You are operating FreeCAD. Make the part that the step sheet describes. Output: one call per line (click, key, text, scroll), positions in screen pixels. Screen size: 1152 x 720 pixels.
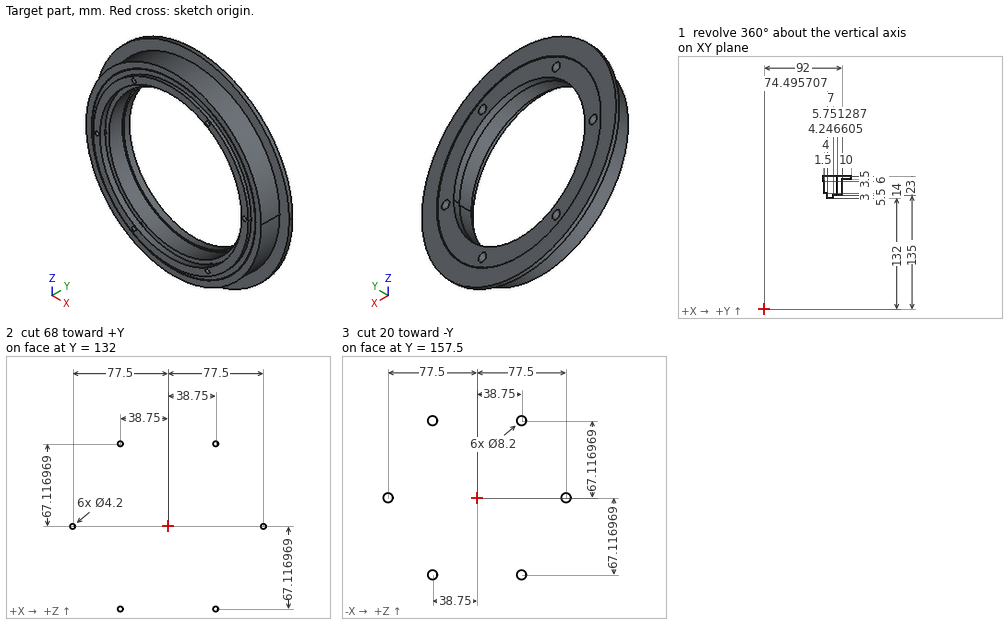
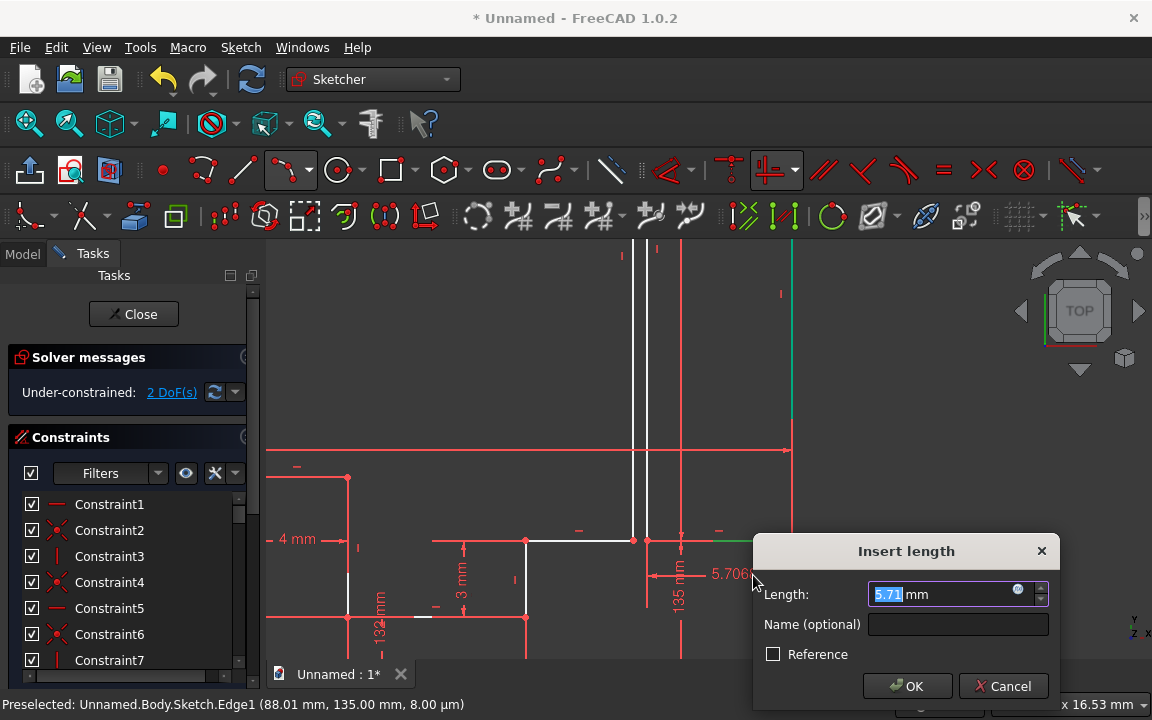
text(5.751287)
key(Return)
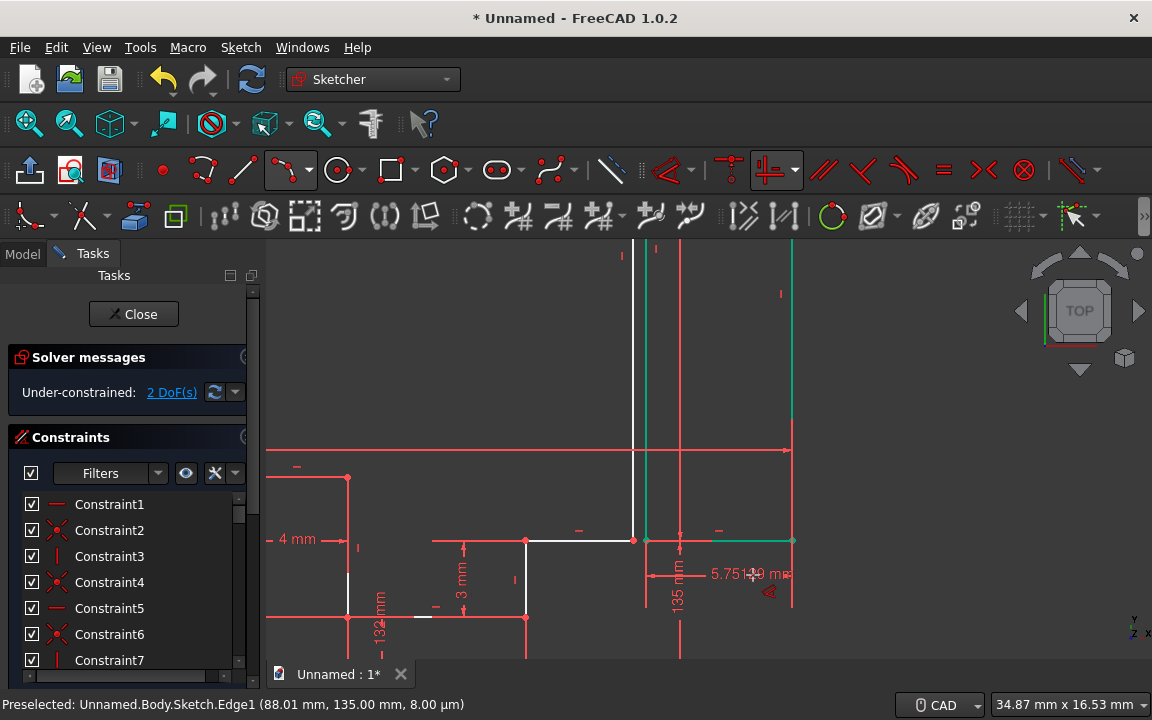
click(558, 541)
click(579, 575)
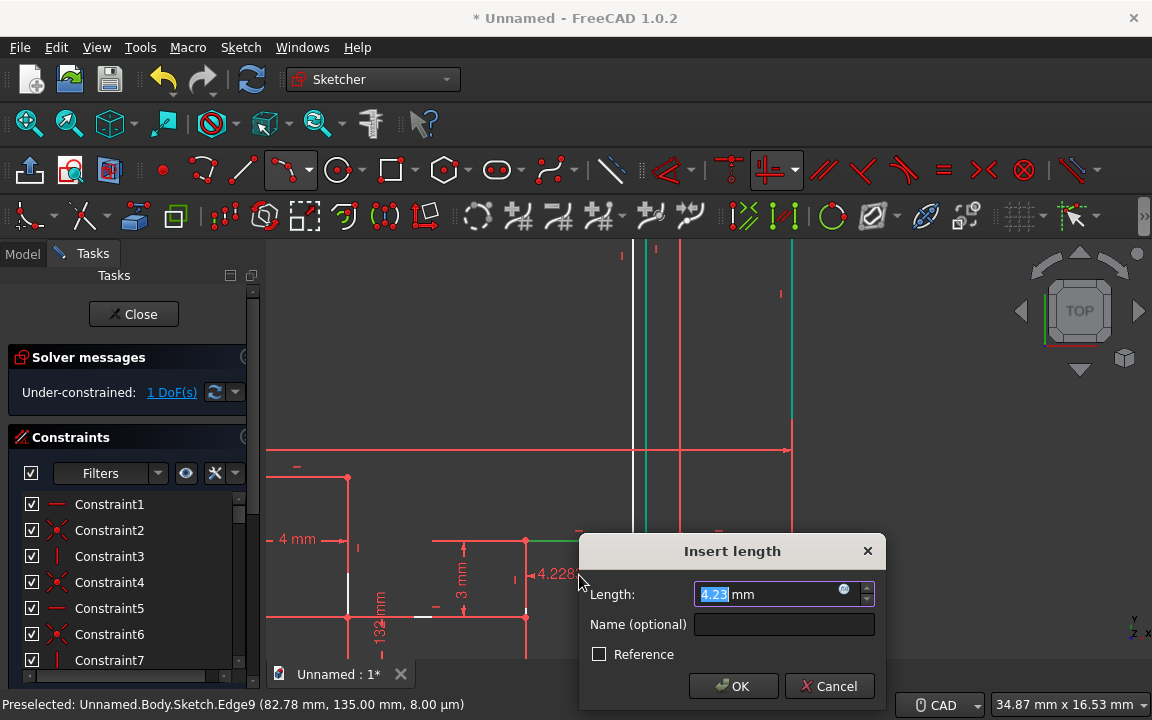
text(4.246605)
key(Return)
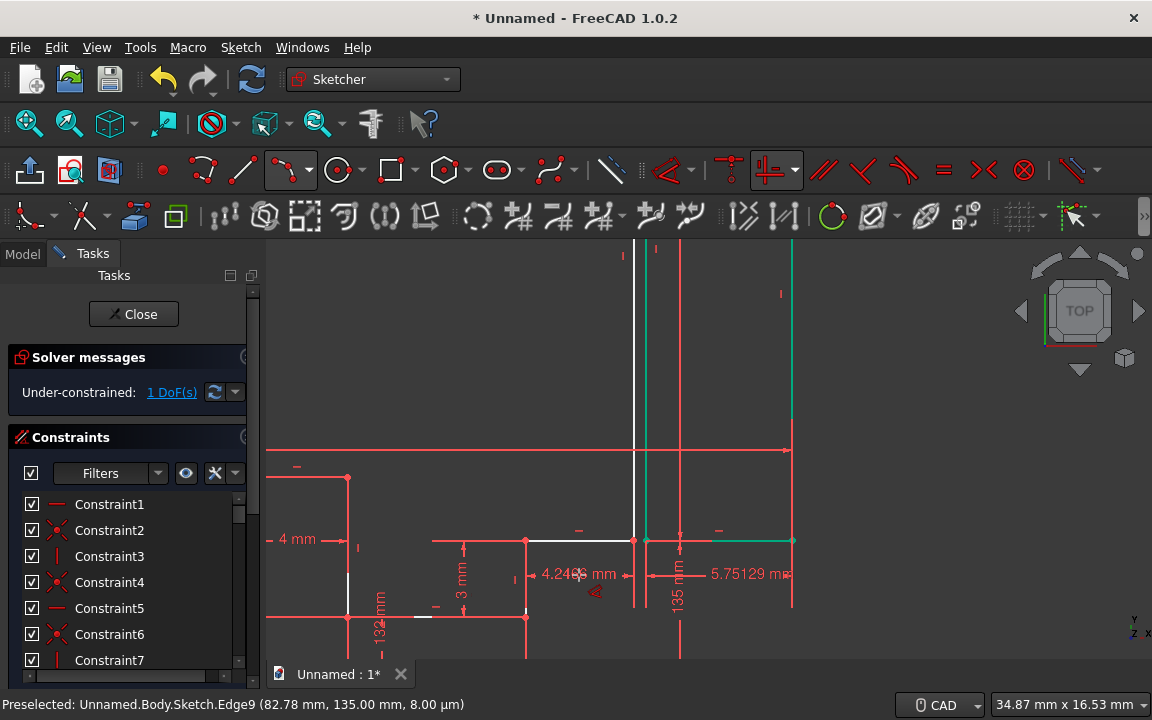
click(348, 617)
click(333, 583)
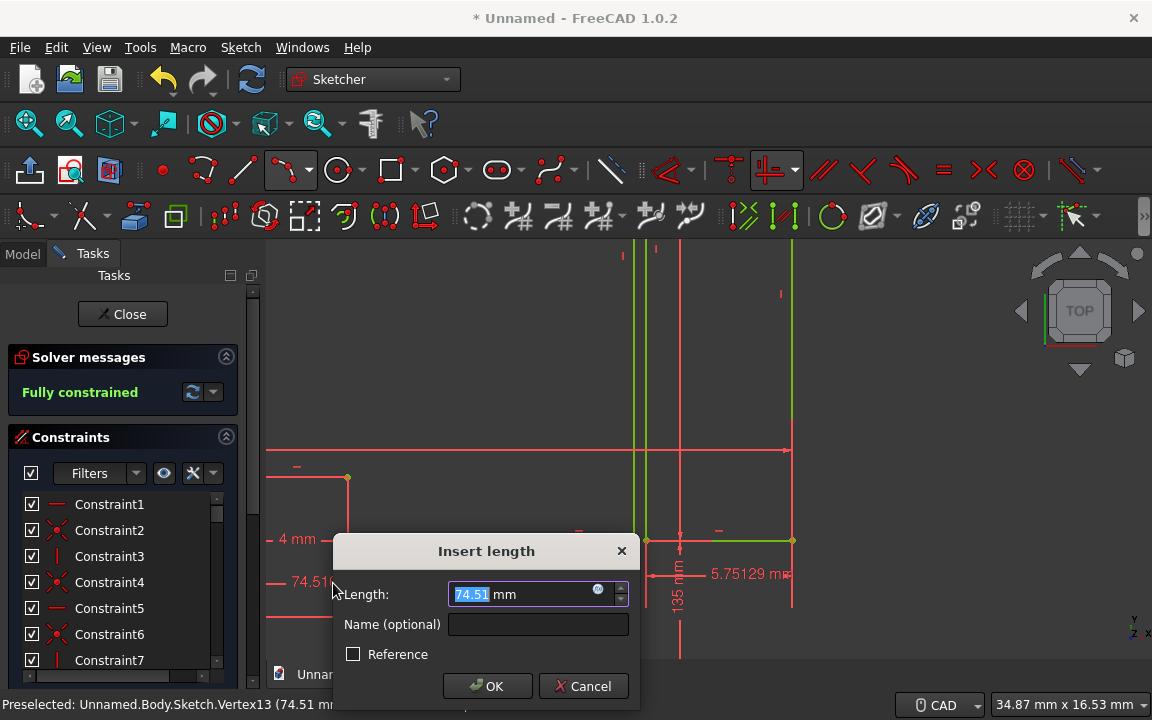
text(74.495707)
key(Return)
key(Escape)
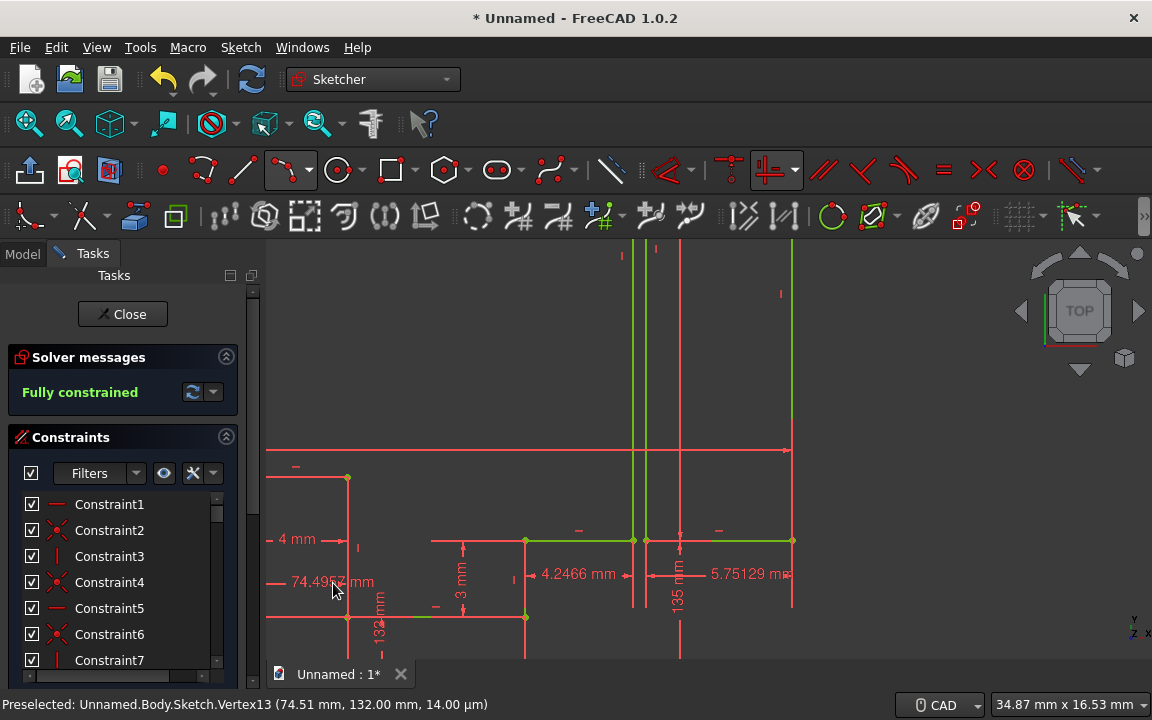
click(123, 314)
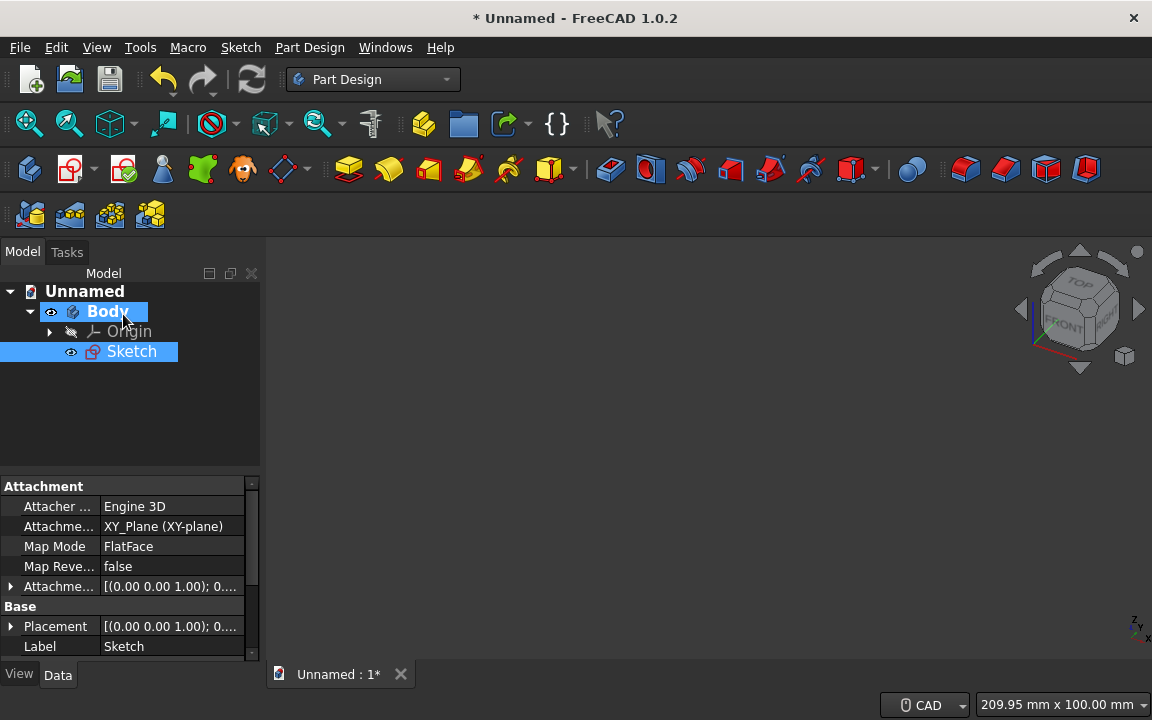
click(390, 170)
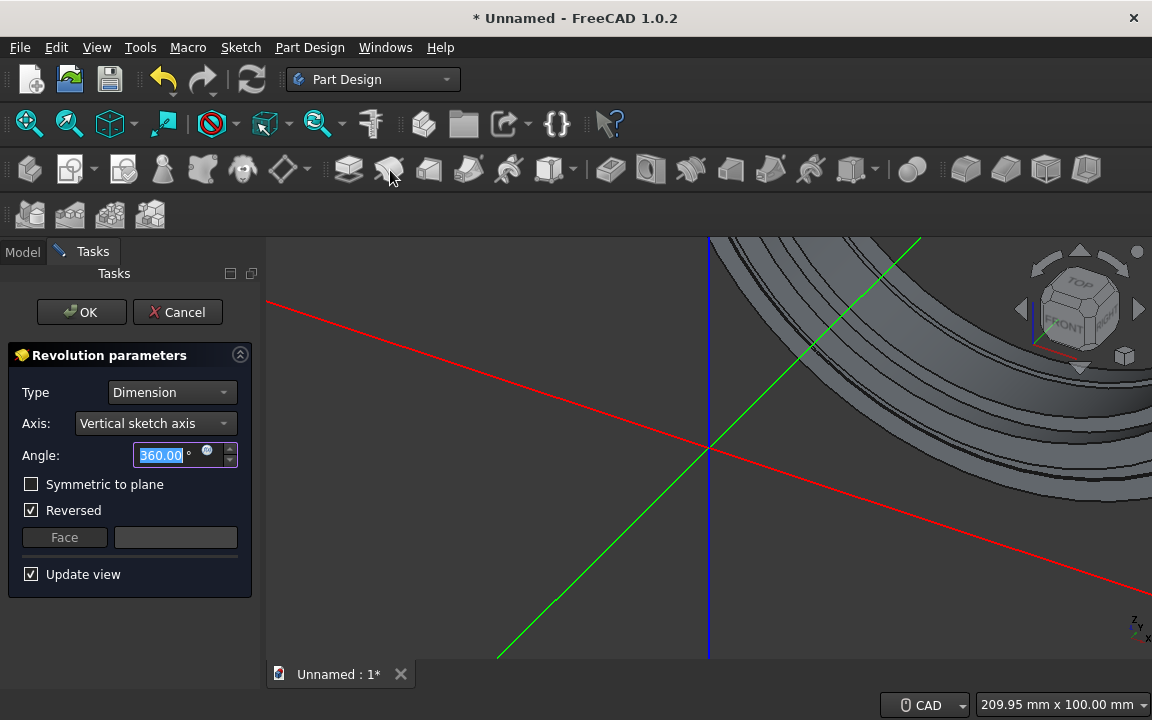
click(82, 312)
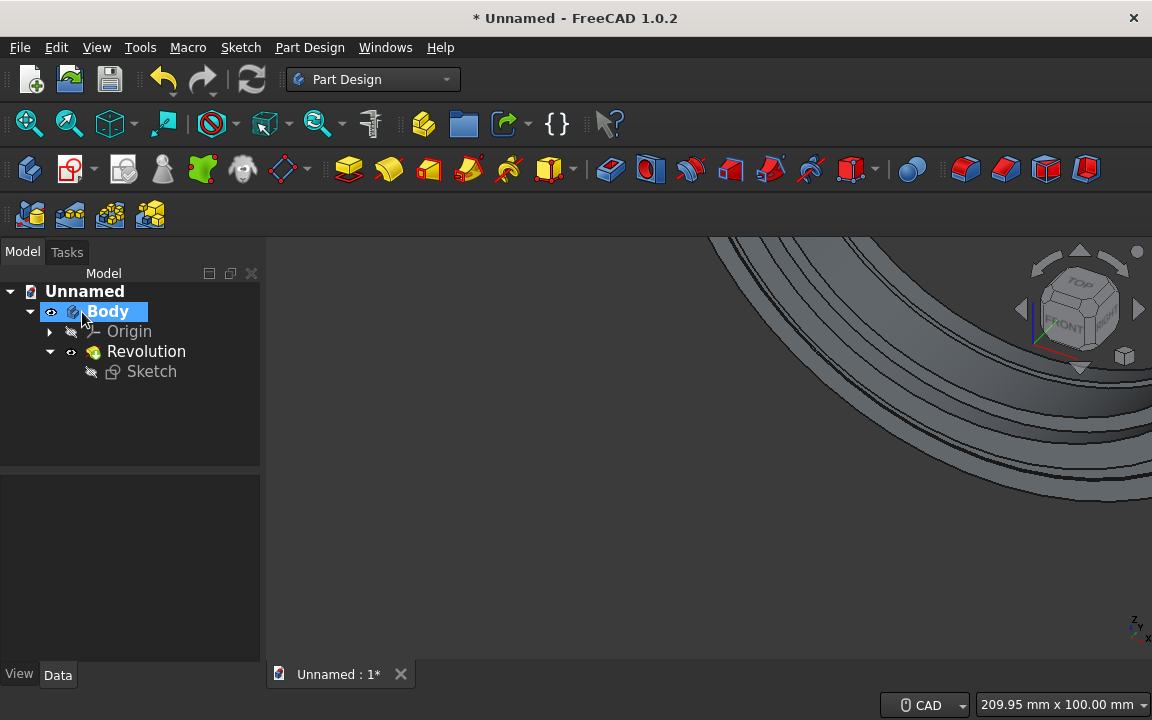
click(30, 124)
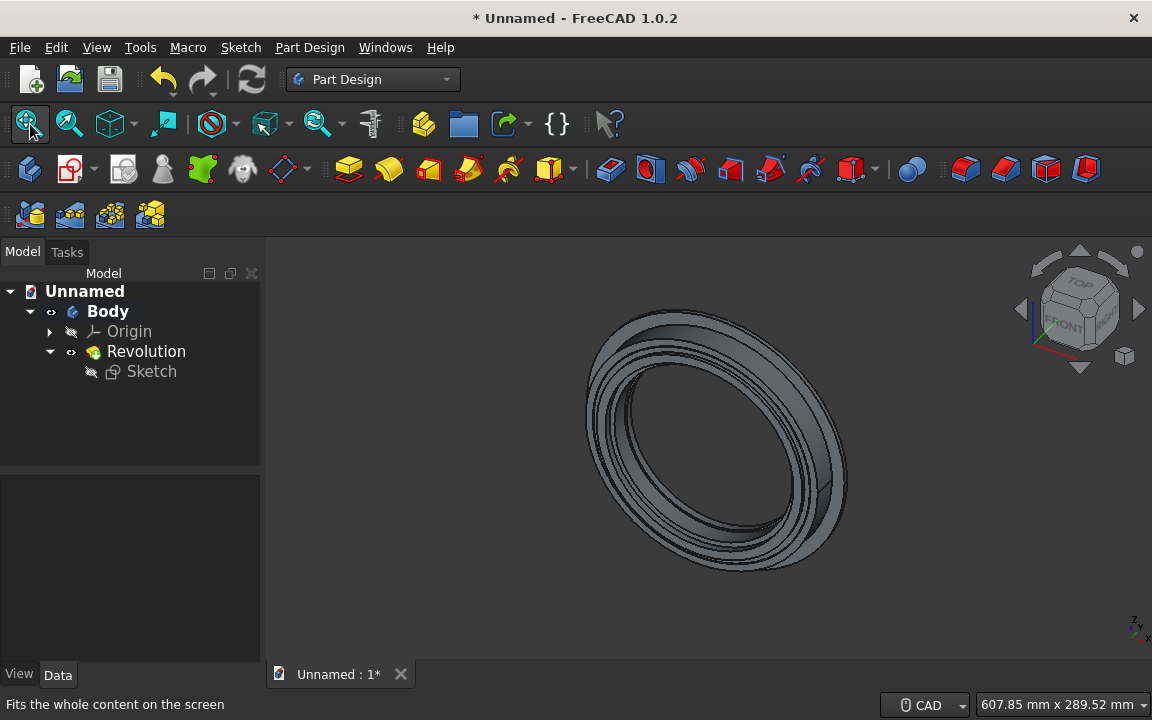
scroll(791, 525, up, 7)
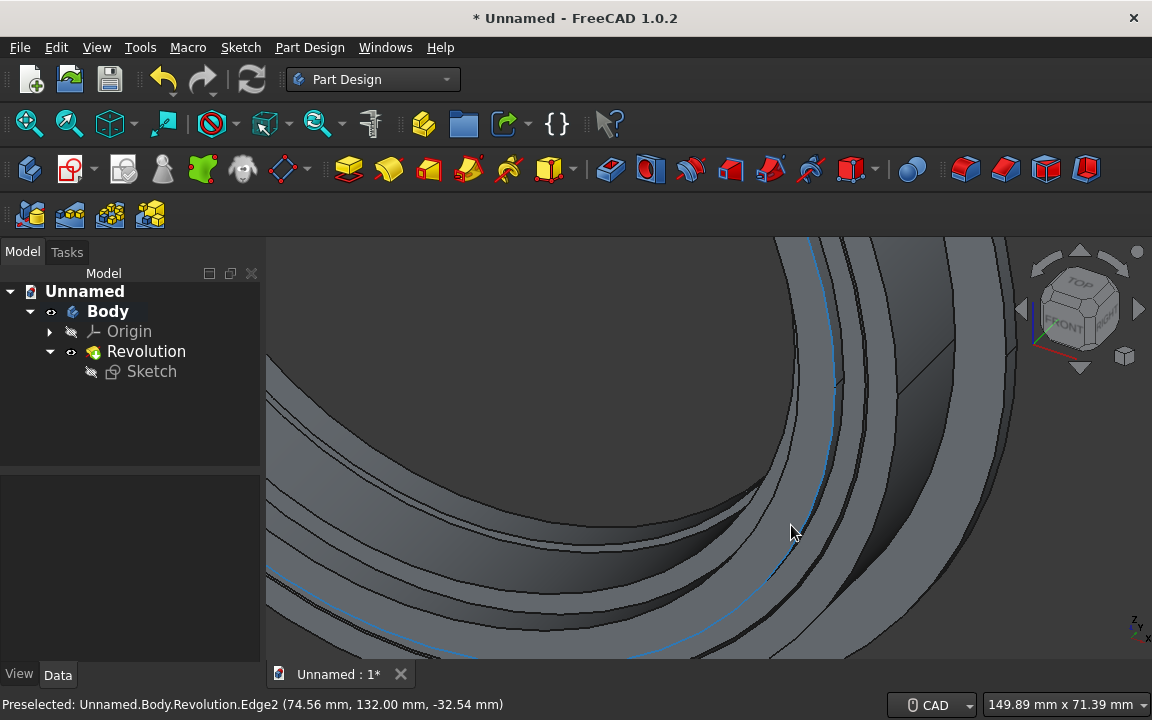
click(788, 525)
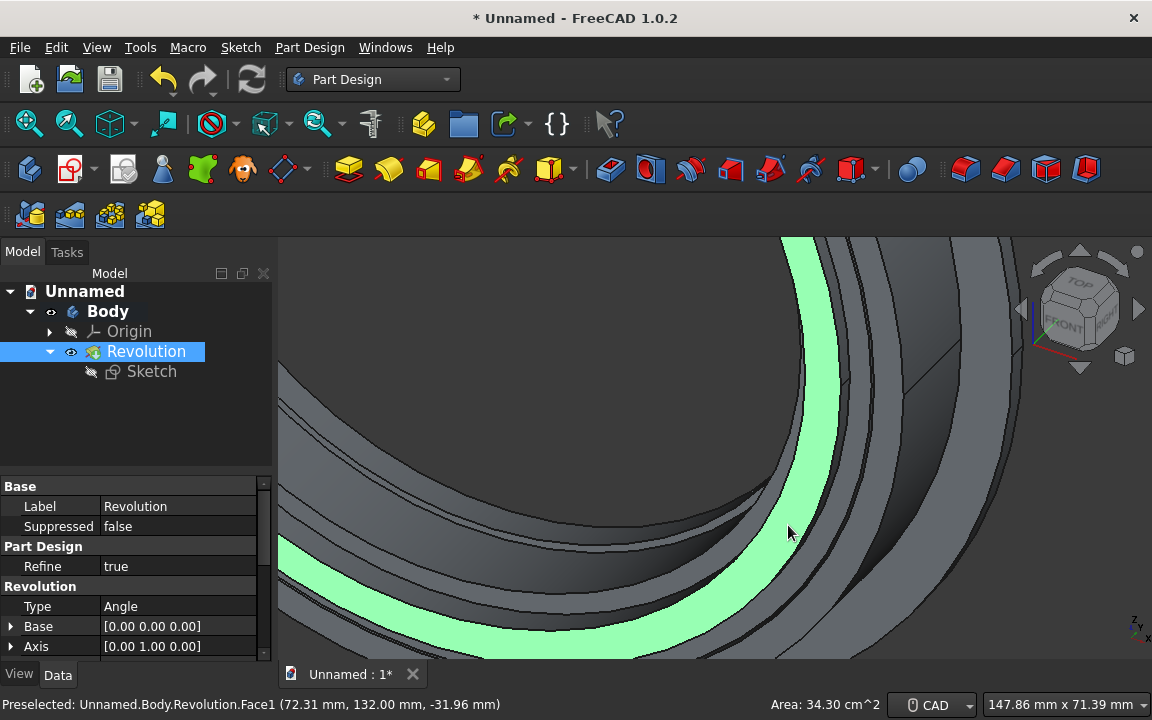
click(70, 170)